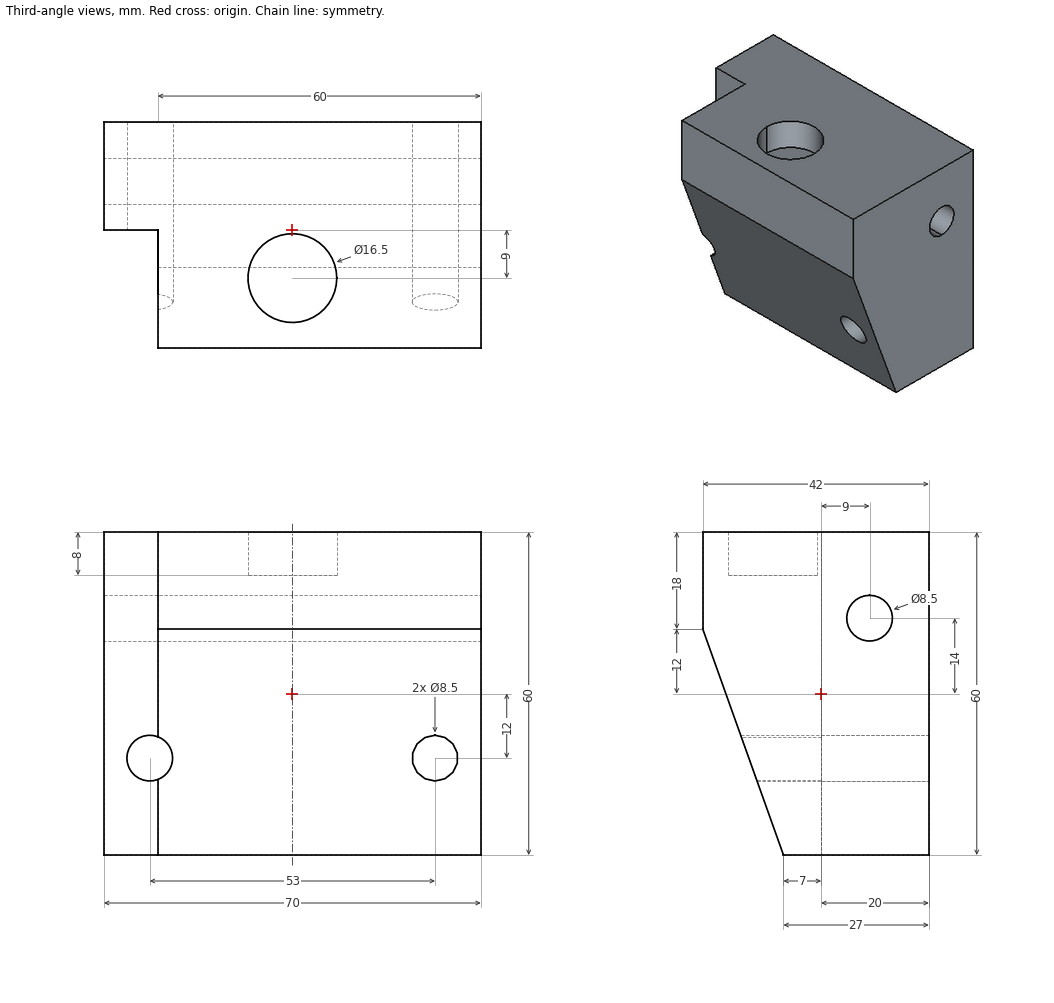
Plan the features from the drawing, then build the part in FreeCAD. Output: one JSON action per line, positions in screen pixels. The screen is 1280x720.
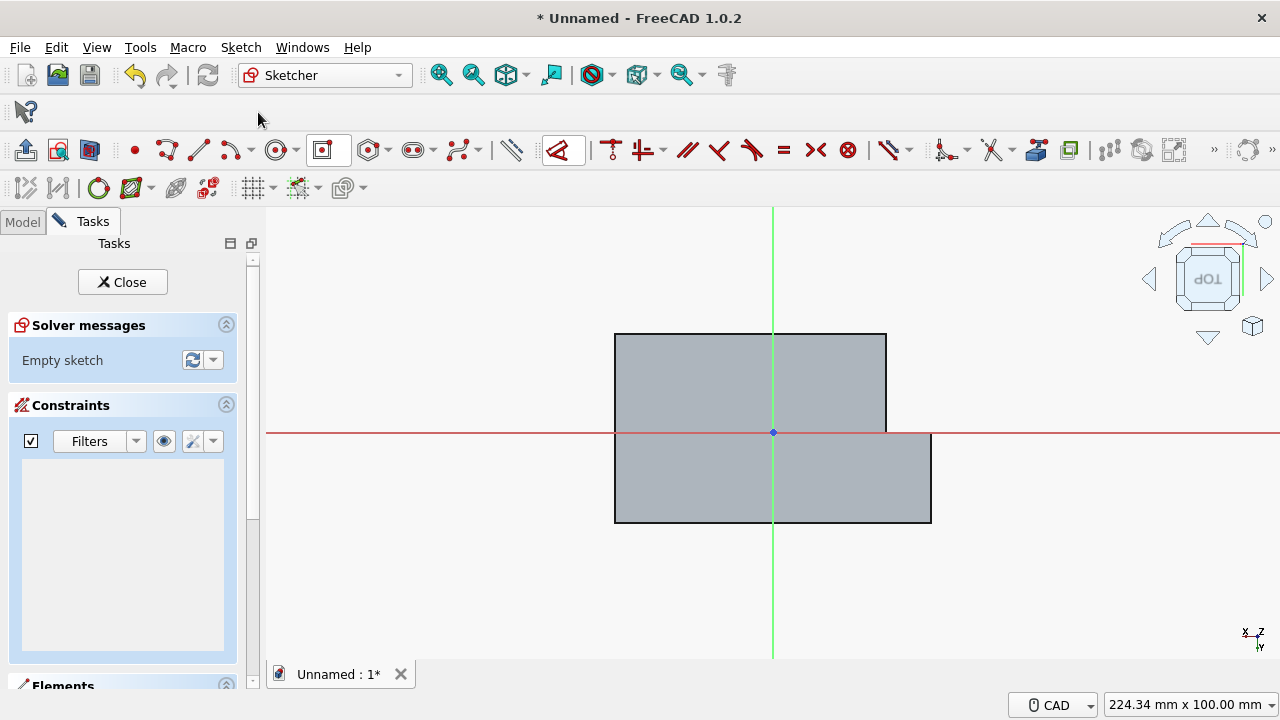
{"action": "scroll", "coordinate": [803, 377], "scroll_direction": "up", "scroll_amount": 6}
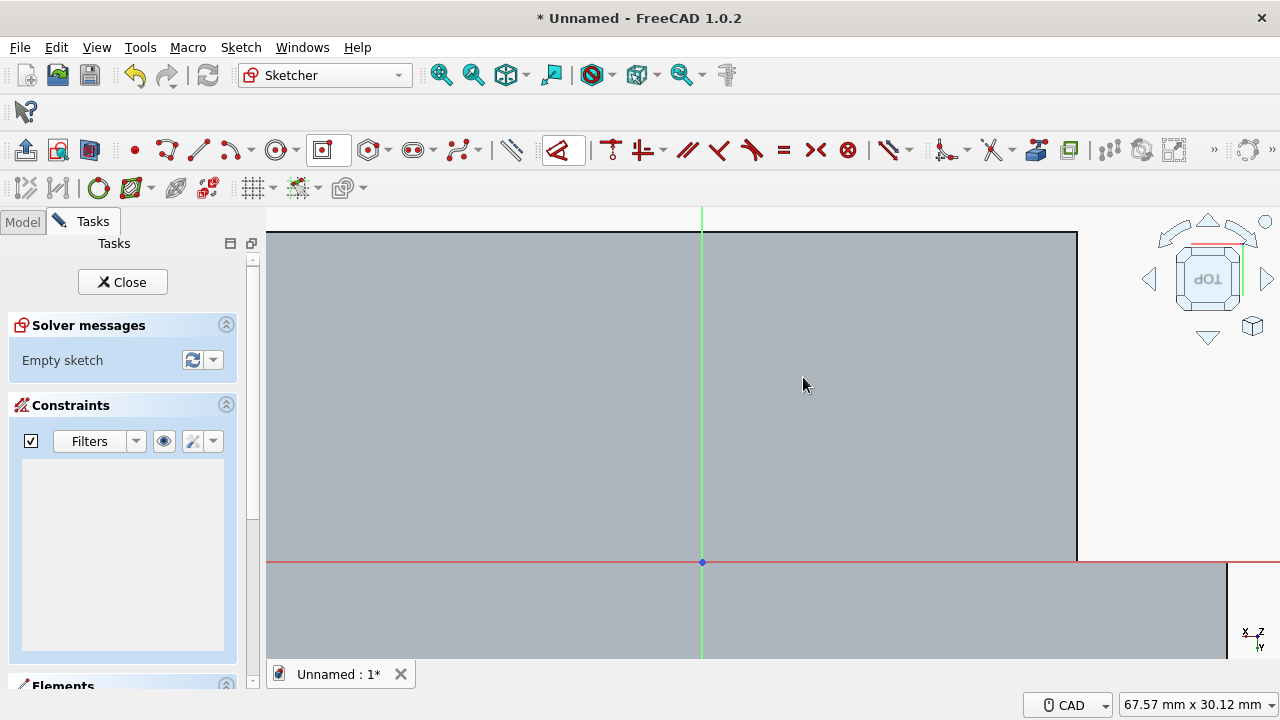
{"action": "key", "text": "g c"}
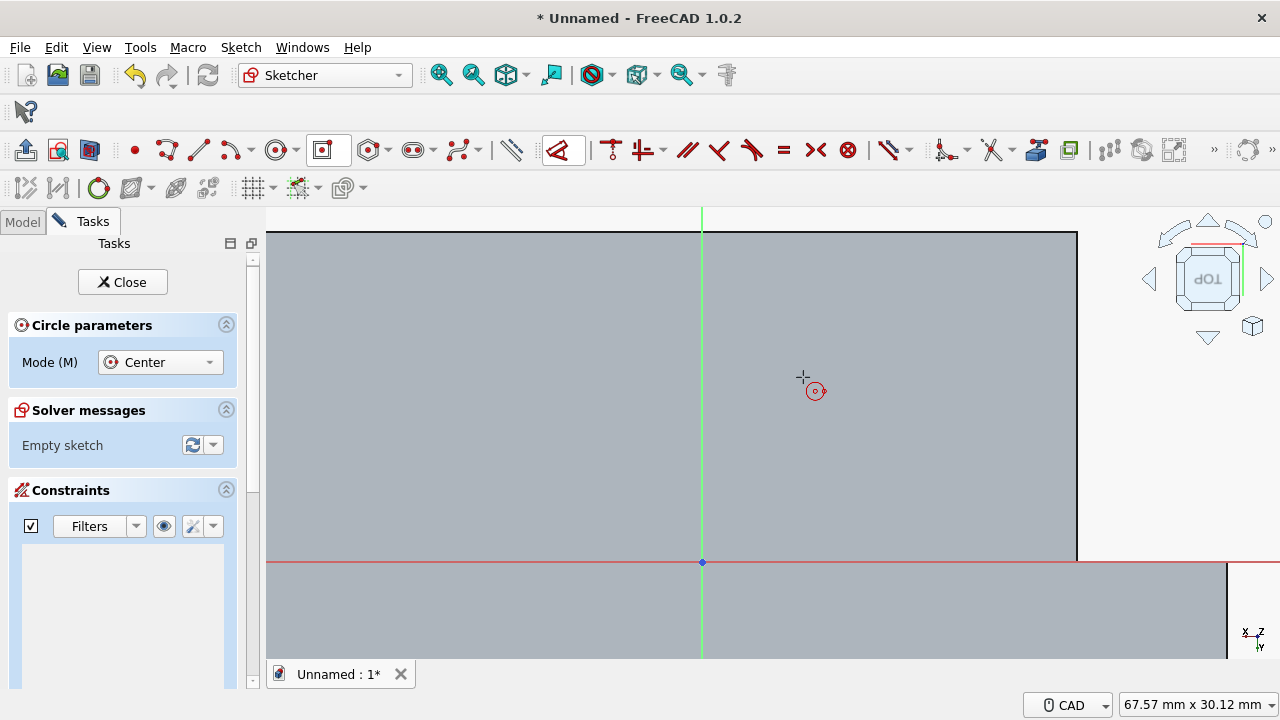
{"action": "left_click", "coordinate": [702, 427]}
{"action": "mouse_move", "coordinate": [790, 339]}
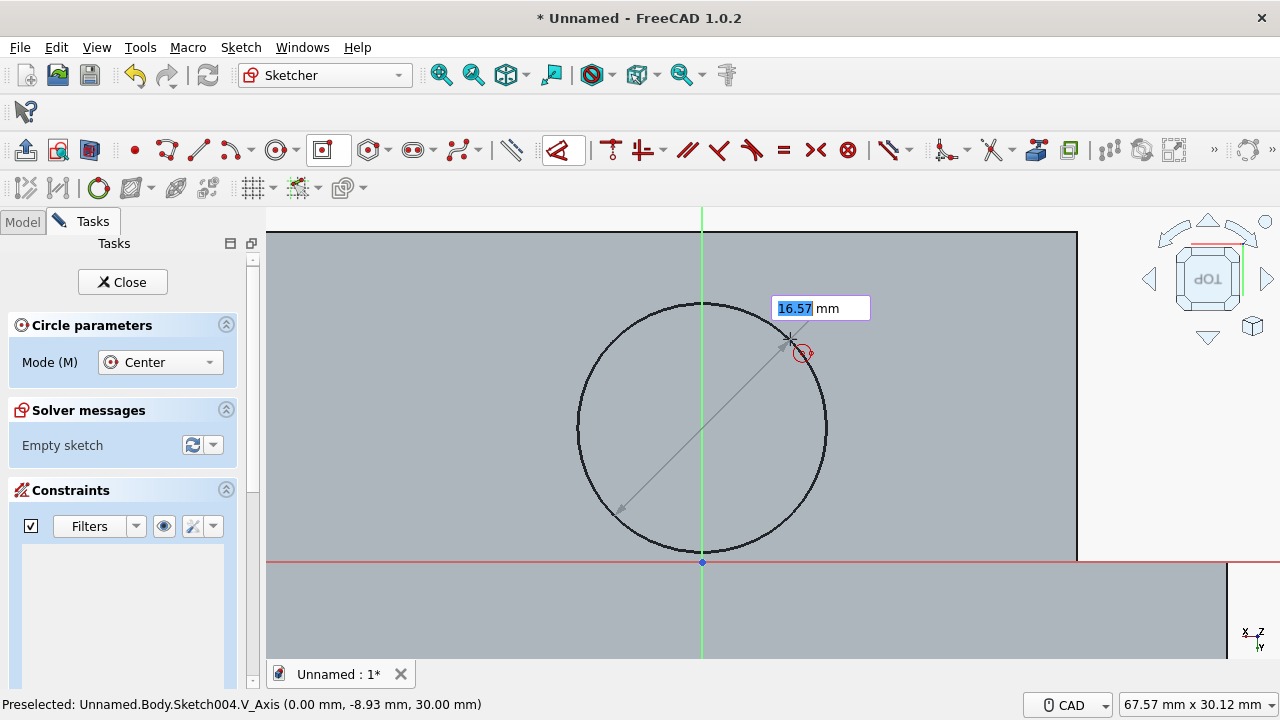
{"action": "type", "text": "16.5"}
{"action": "key", "text": "Return"}
{"action": "key", "text": "Escape"}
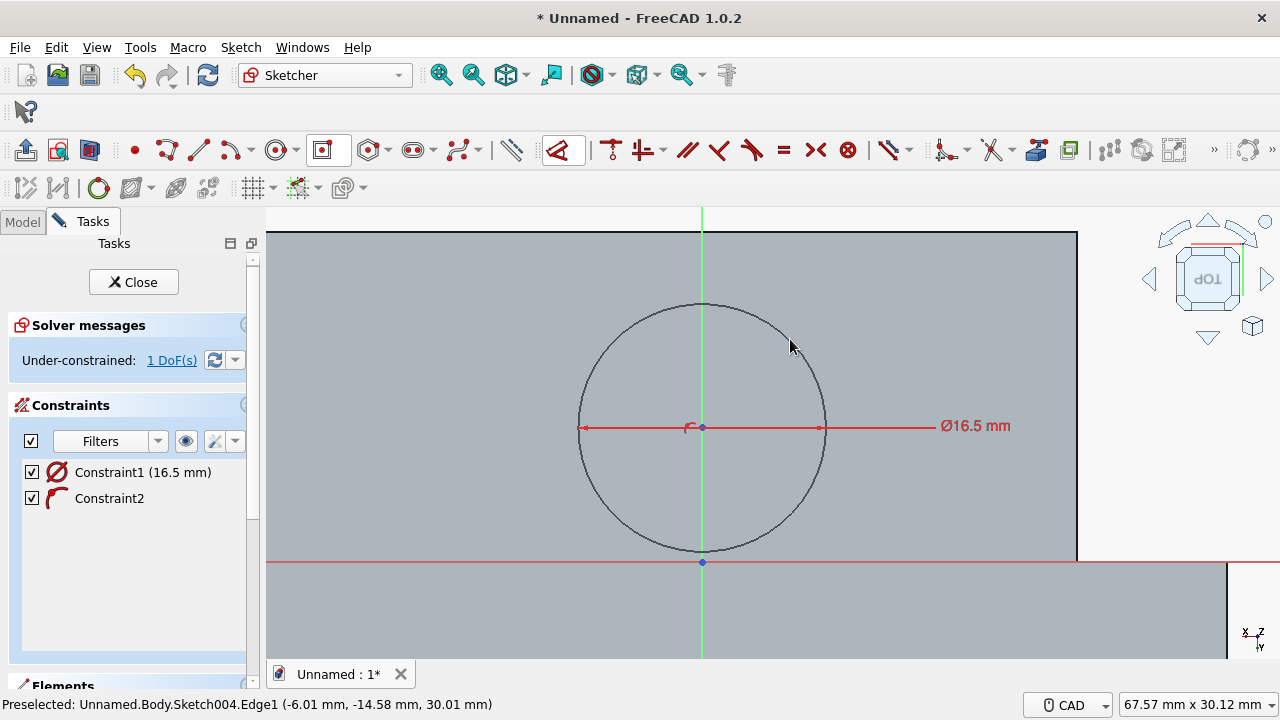
{"action": "left_click", "coordinate": [702, 428]}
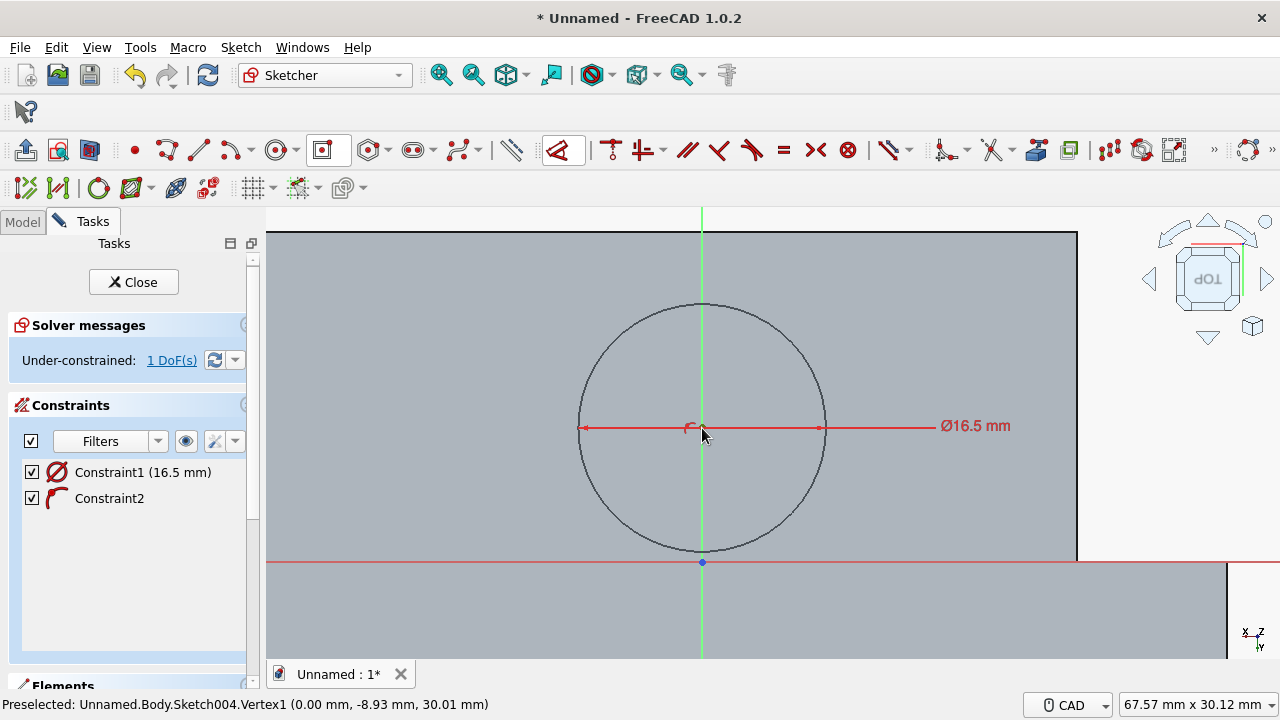
{"action": "key", "text": "i"}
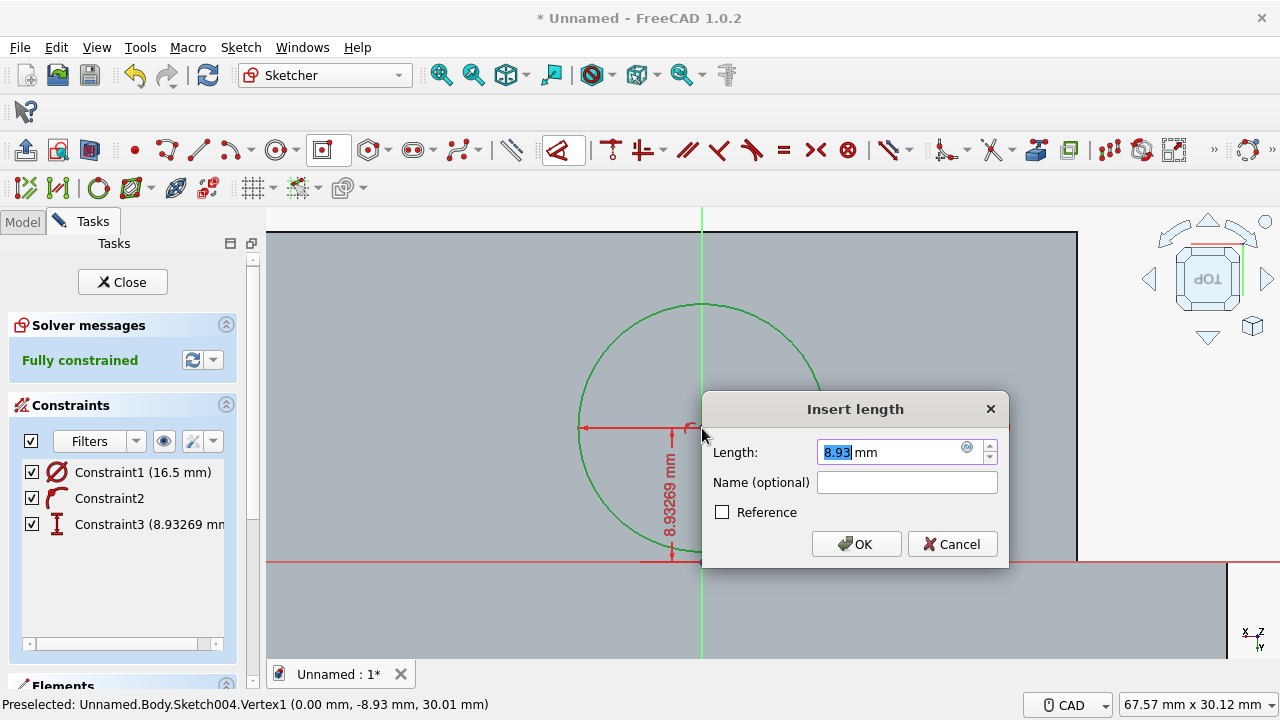
{"action": "type", "text": "9"}
{"action": "key", "text": "Return"}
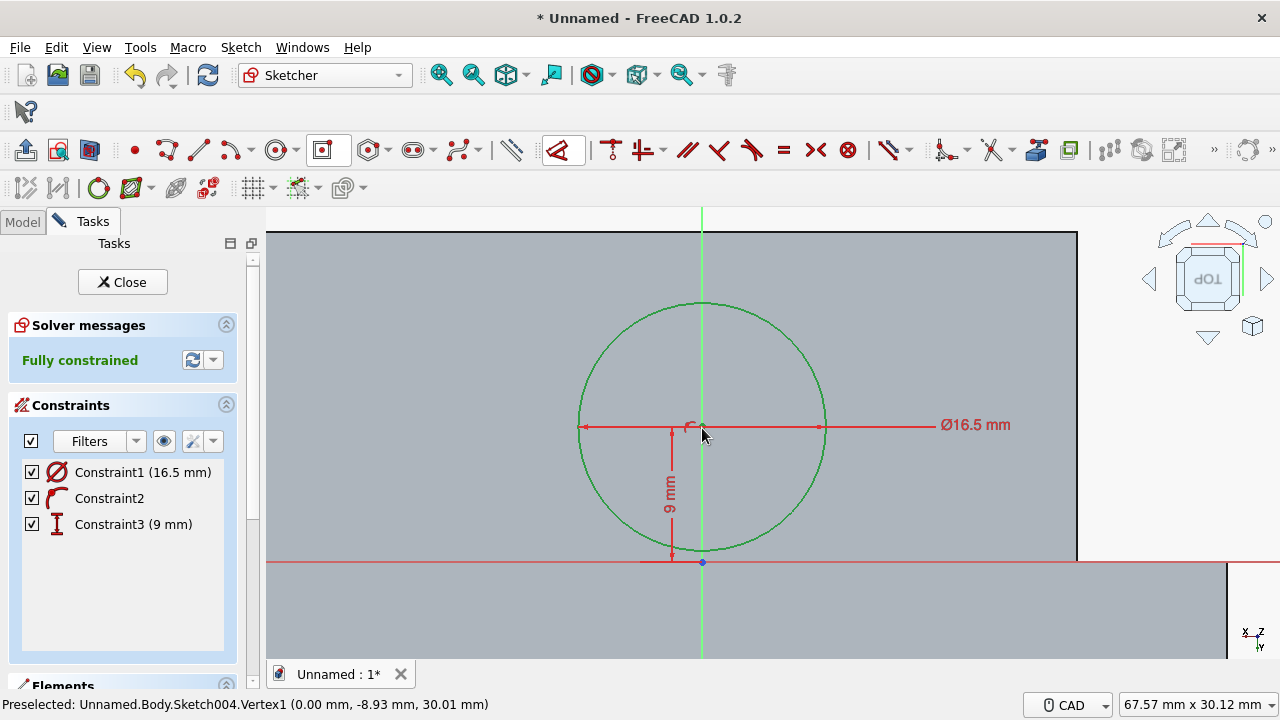
{"action": "left_click", "coordinate": [123, 282]}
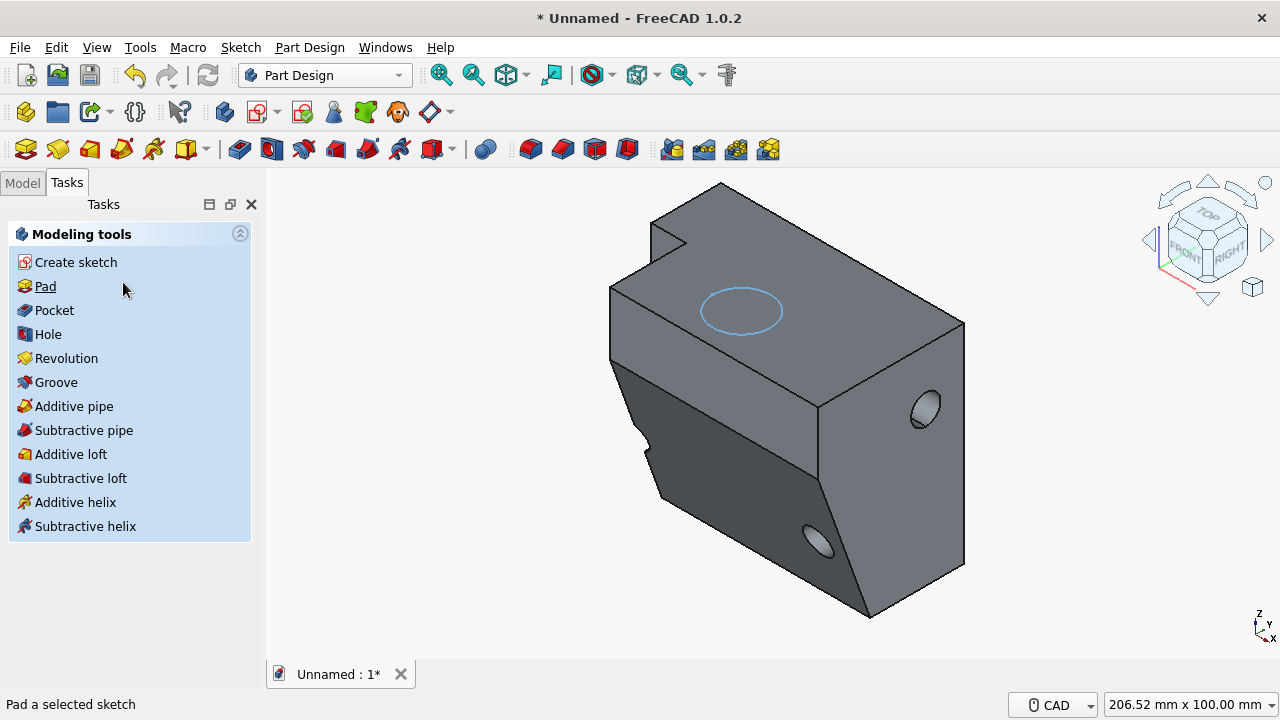
{"action": "left_click", "coordinate": [240, 150]}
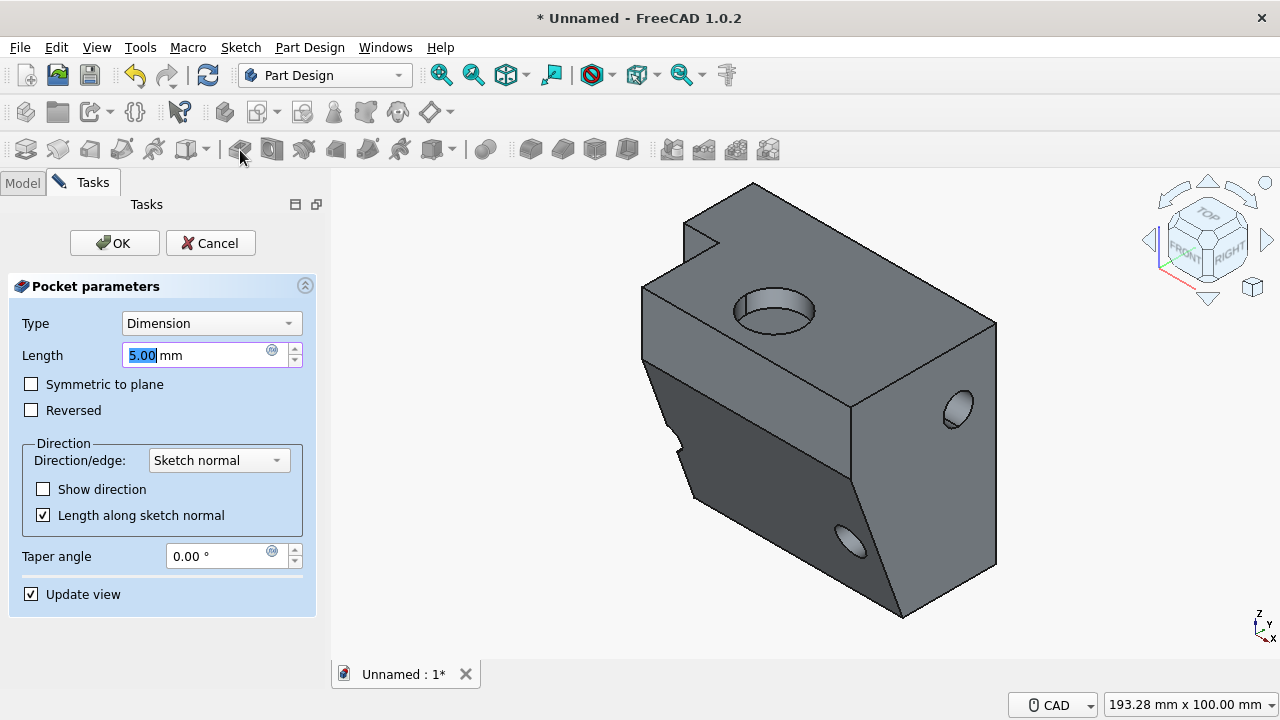
{"action": "type", "text": "8"}
{"action": "key", "text": "Tab"}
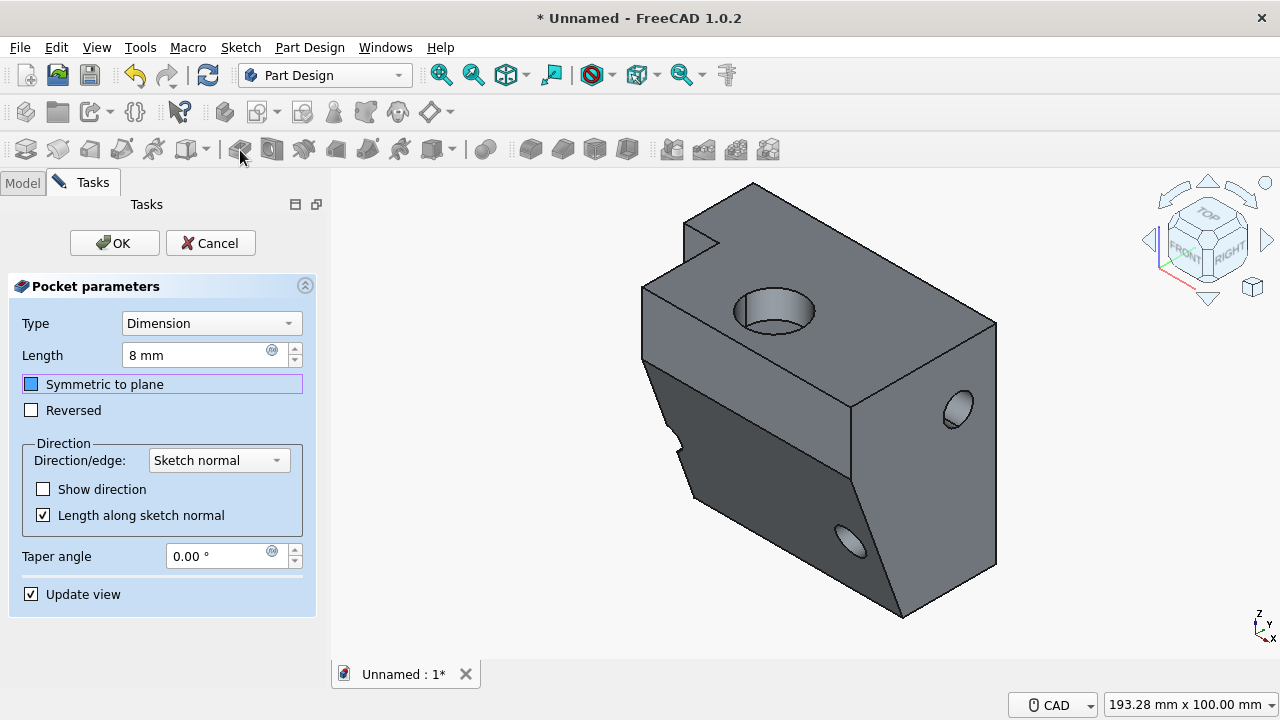
{"action": "left_click", "coordinate": [115, 243]}